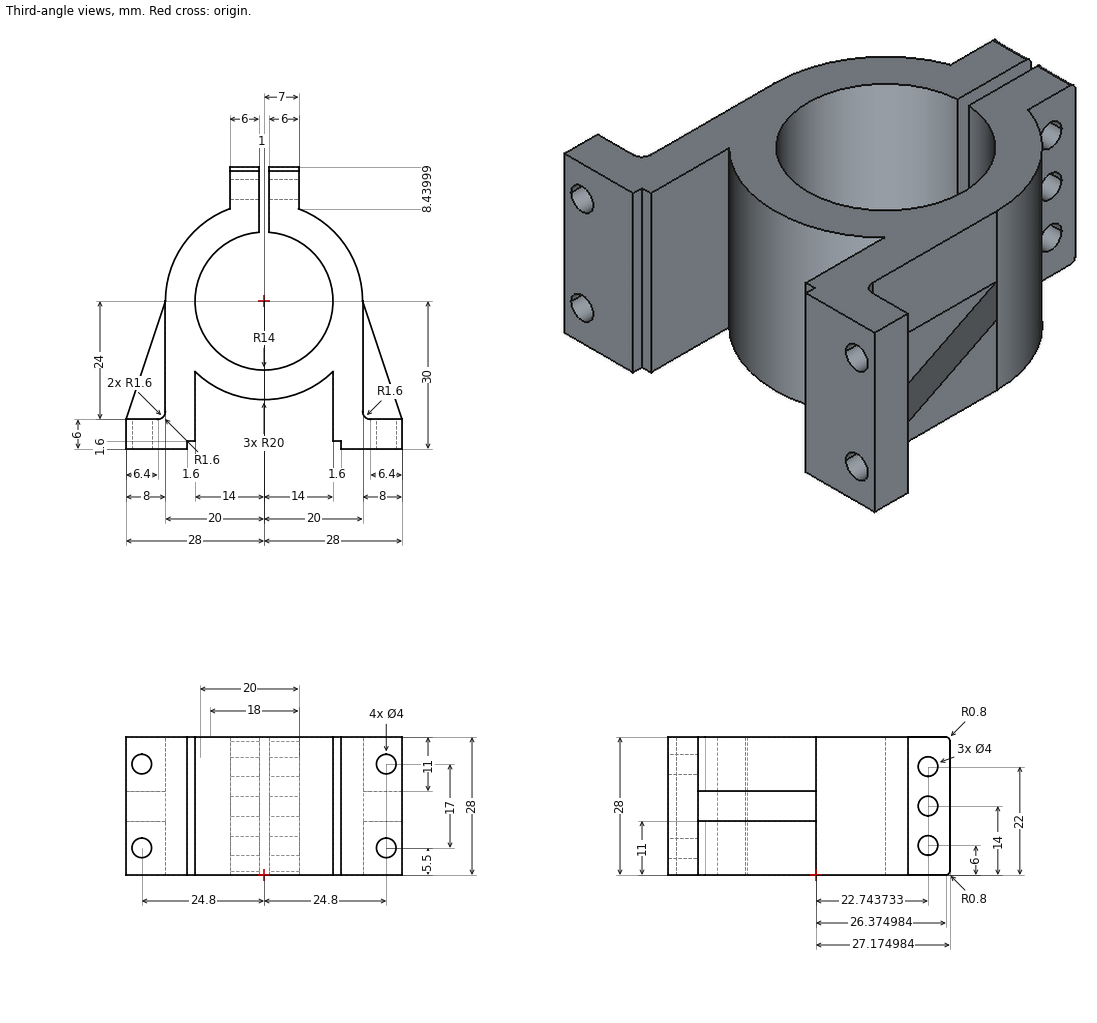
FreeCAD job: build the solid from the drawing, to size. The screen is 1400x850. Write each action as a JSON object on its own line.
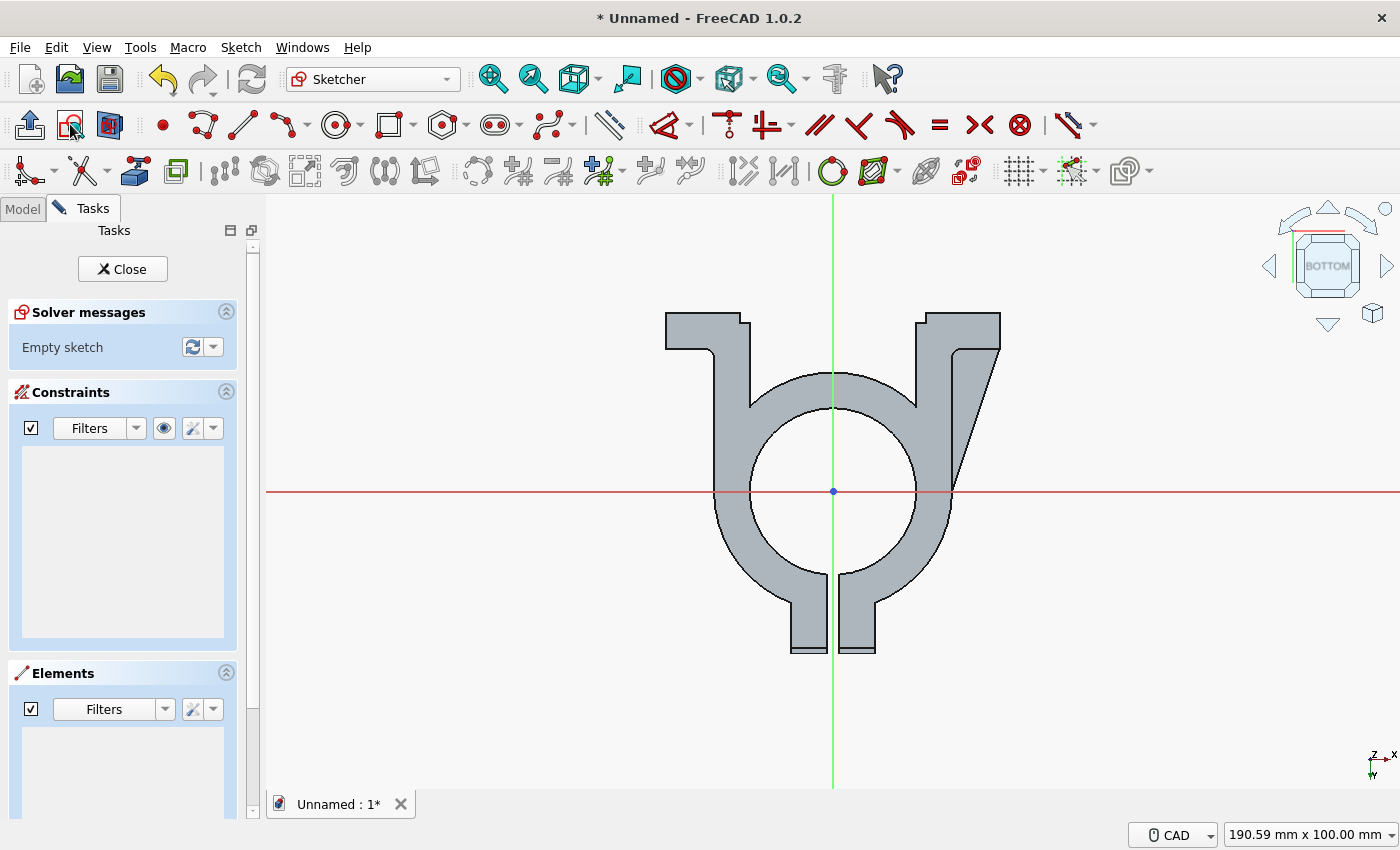
{"action": "scroll", "coordinate": [741, 379], "scroll_direction": "up", "scroll_amount": 5}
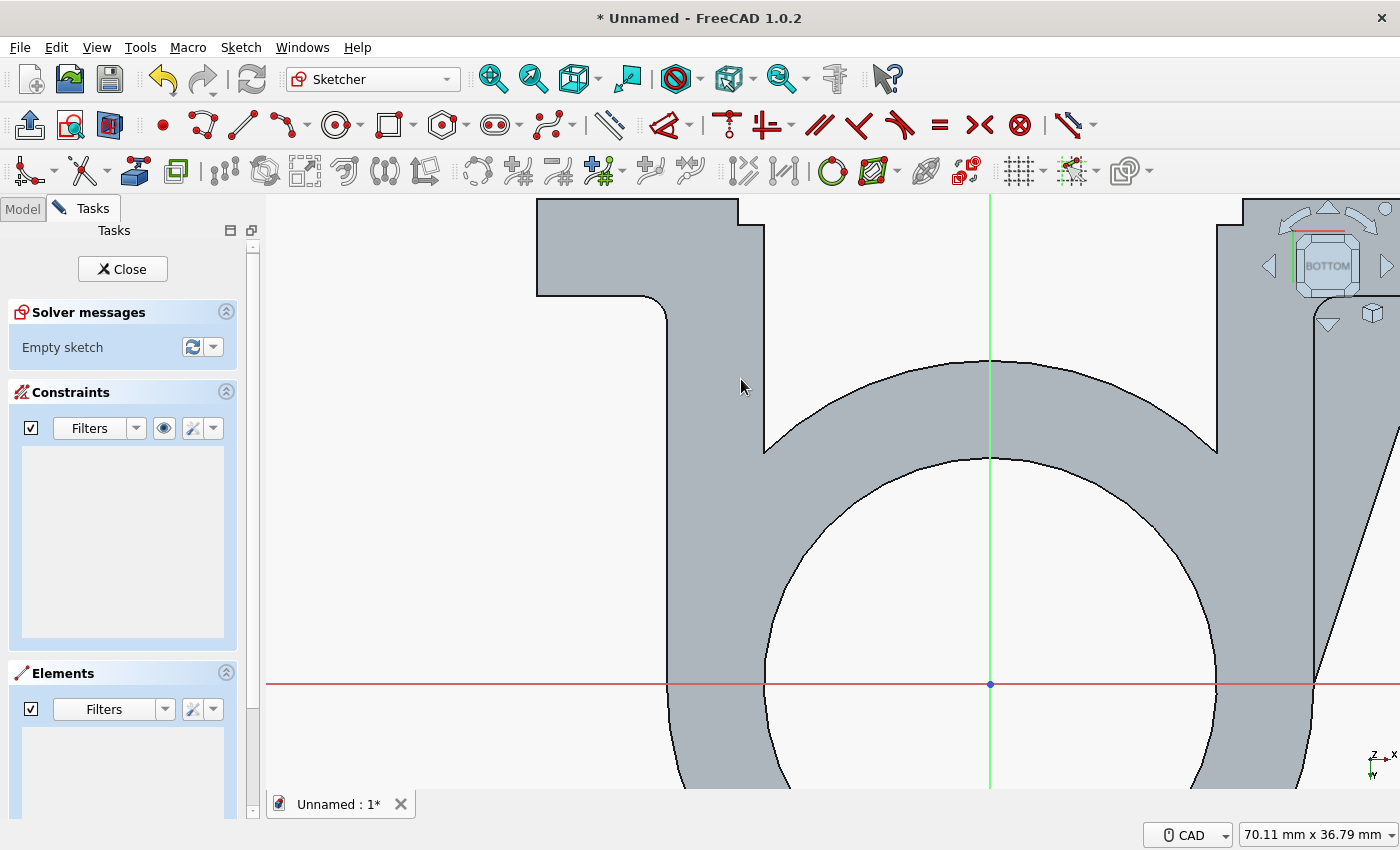
{"action": "left_click", "coordinate": [204, 126]}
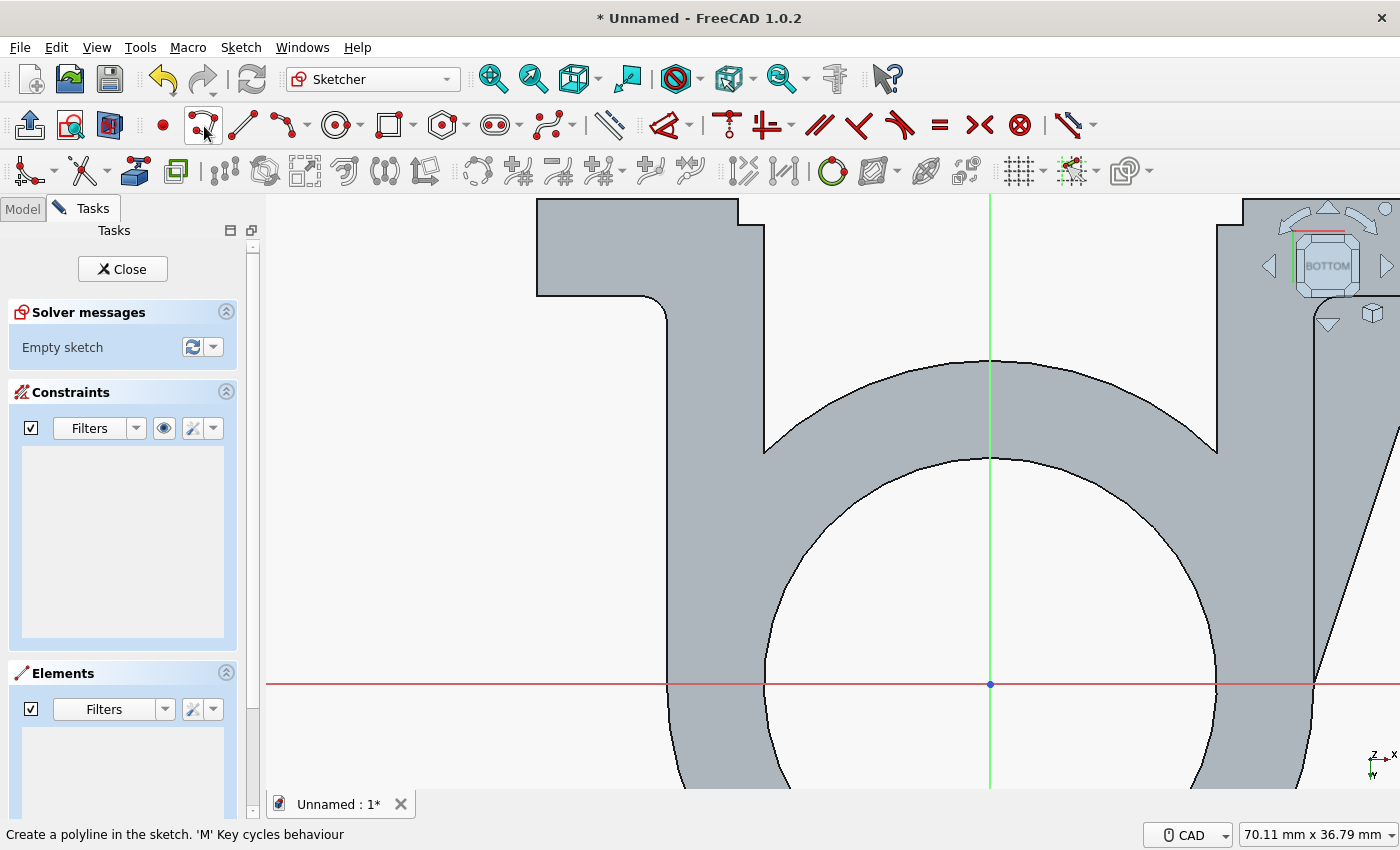
{"action": "left_click", "coordinate": [641, 296]}
{"action": "left_click", "coordinate": [537, 296]}
{"action": "left_click", "coordinate": [667, 684]}
{"action": "left_click", "coordinate": [667, 322]}
{"action": "right_click", "coordinate": [667, 322]}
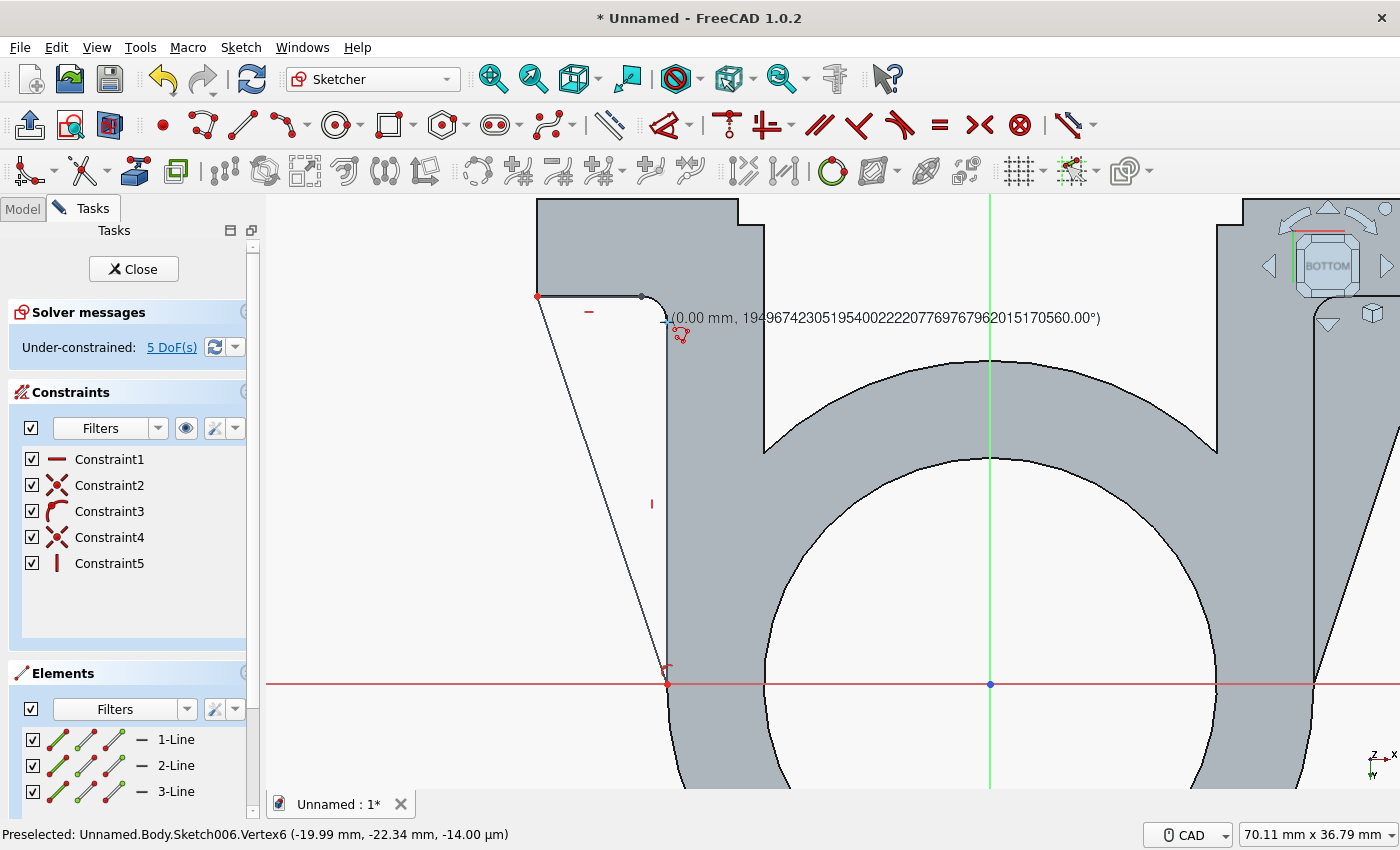
{"action": "left_click", "coordinate": [284, 126]}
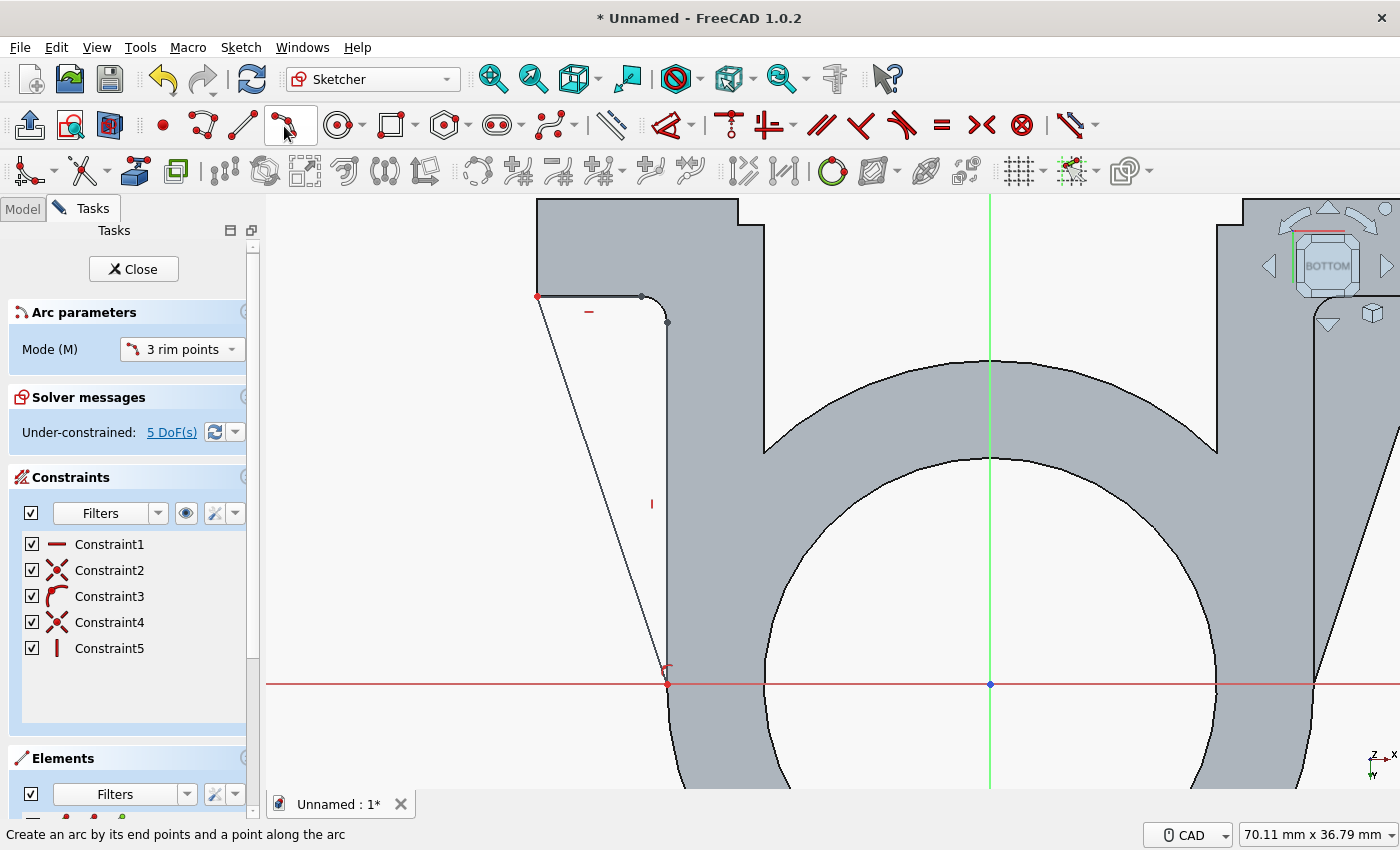
{"action": "left_click", "coordinate": [667, 323]}
{"action": "left_click", "coordinate": [641, 297]}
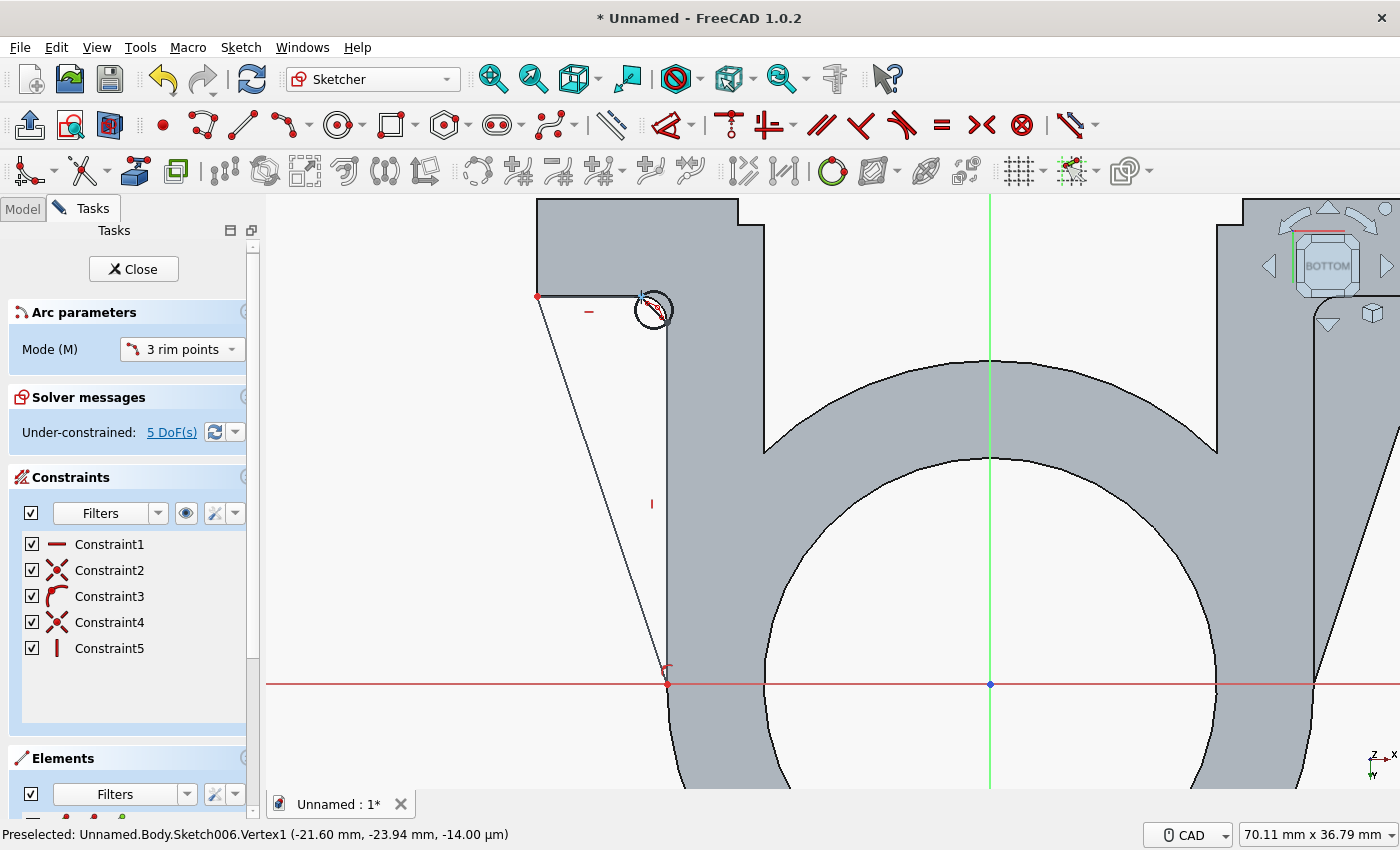
{"action": "scroll", "coordinate": [659, 304], "scroll_direction": "up", "scroll_amount": 4}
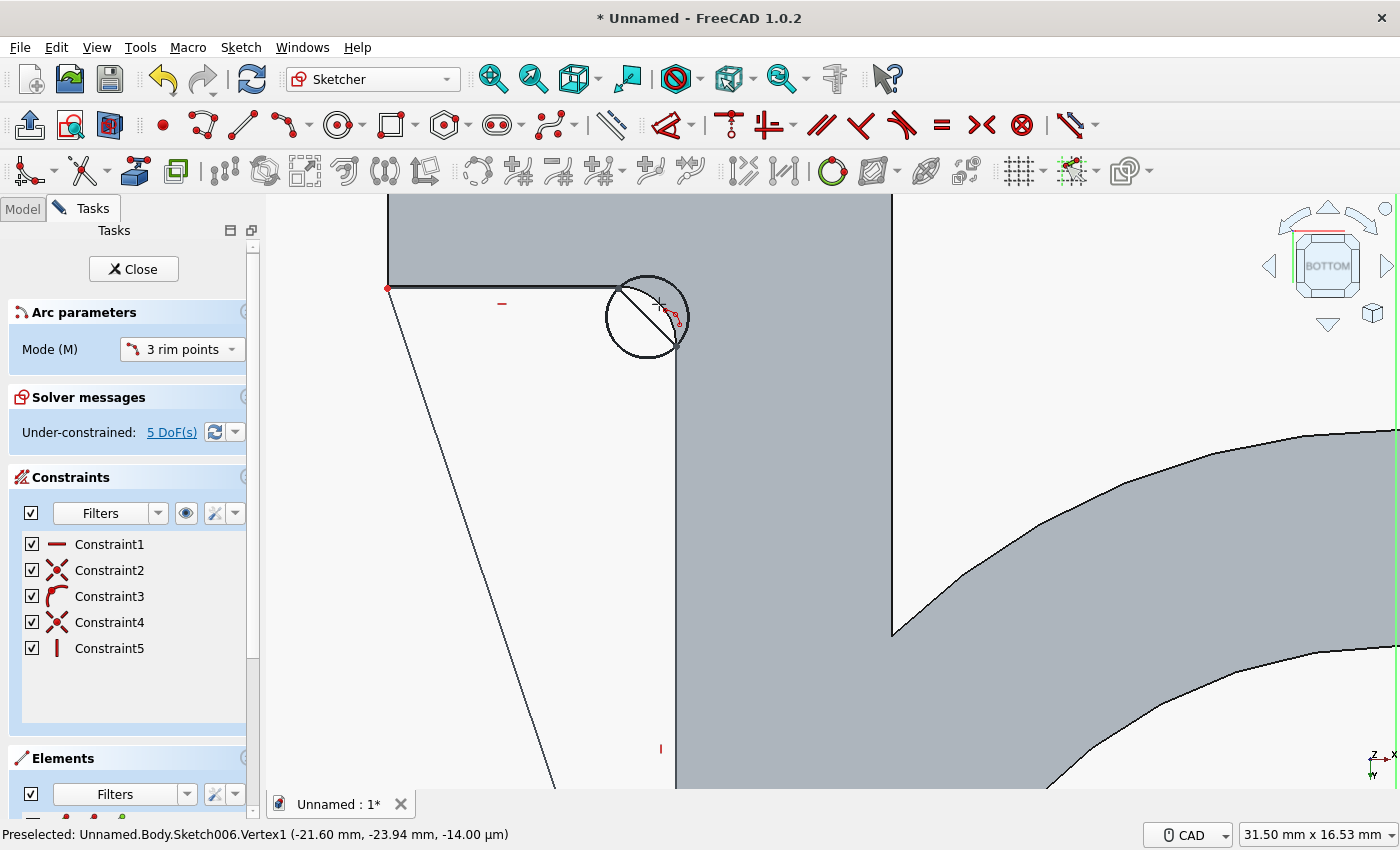
{"action": "left_click", "coordinate": [659, 303]}
{"action": "key", "text": "Escape"}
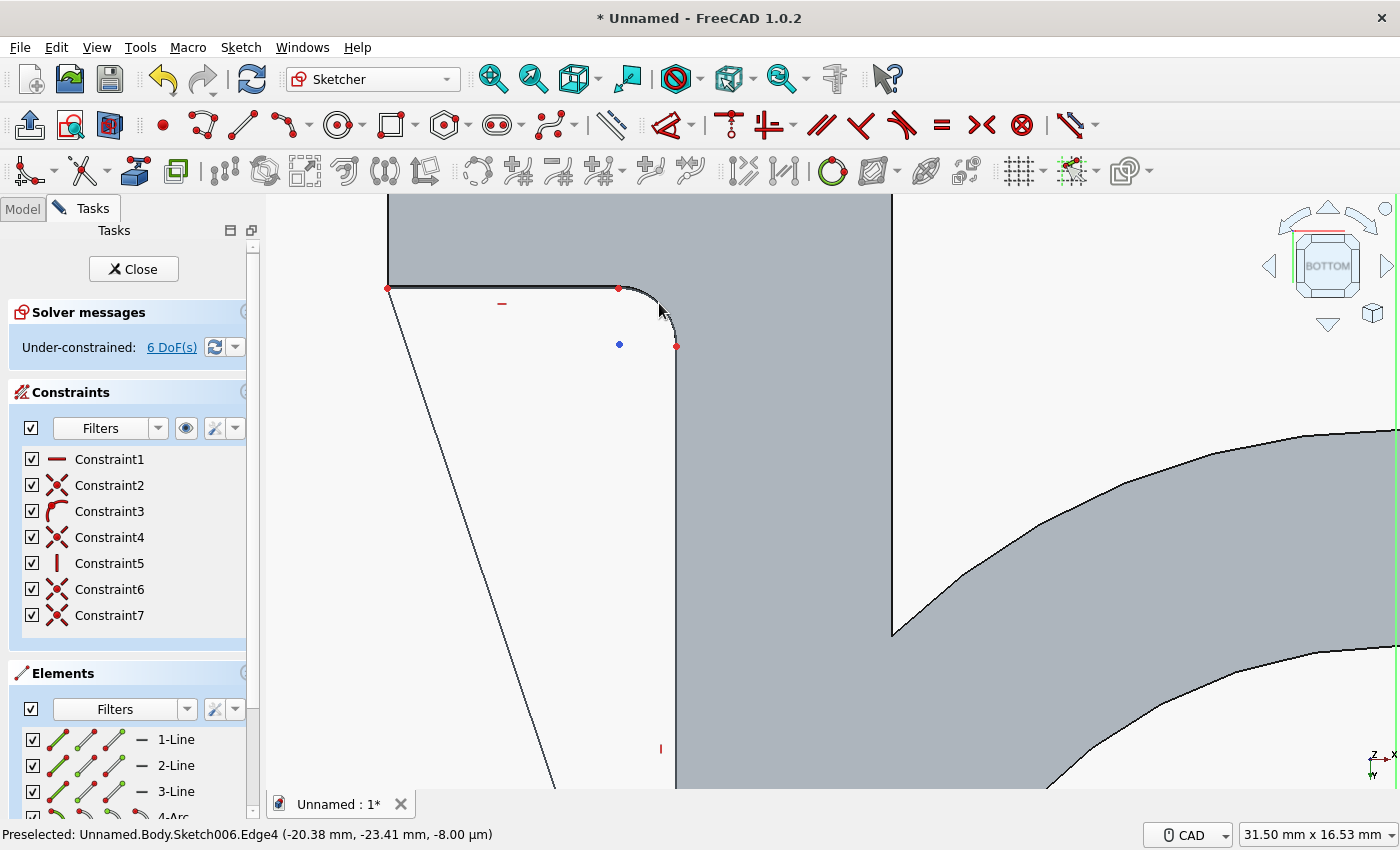
{"action": "left_click", "coordinate": [549, 288]}